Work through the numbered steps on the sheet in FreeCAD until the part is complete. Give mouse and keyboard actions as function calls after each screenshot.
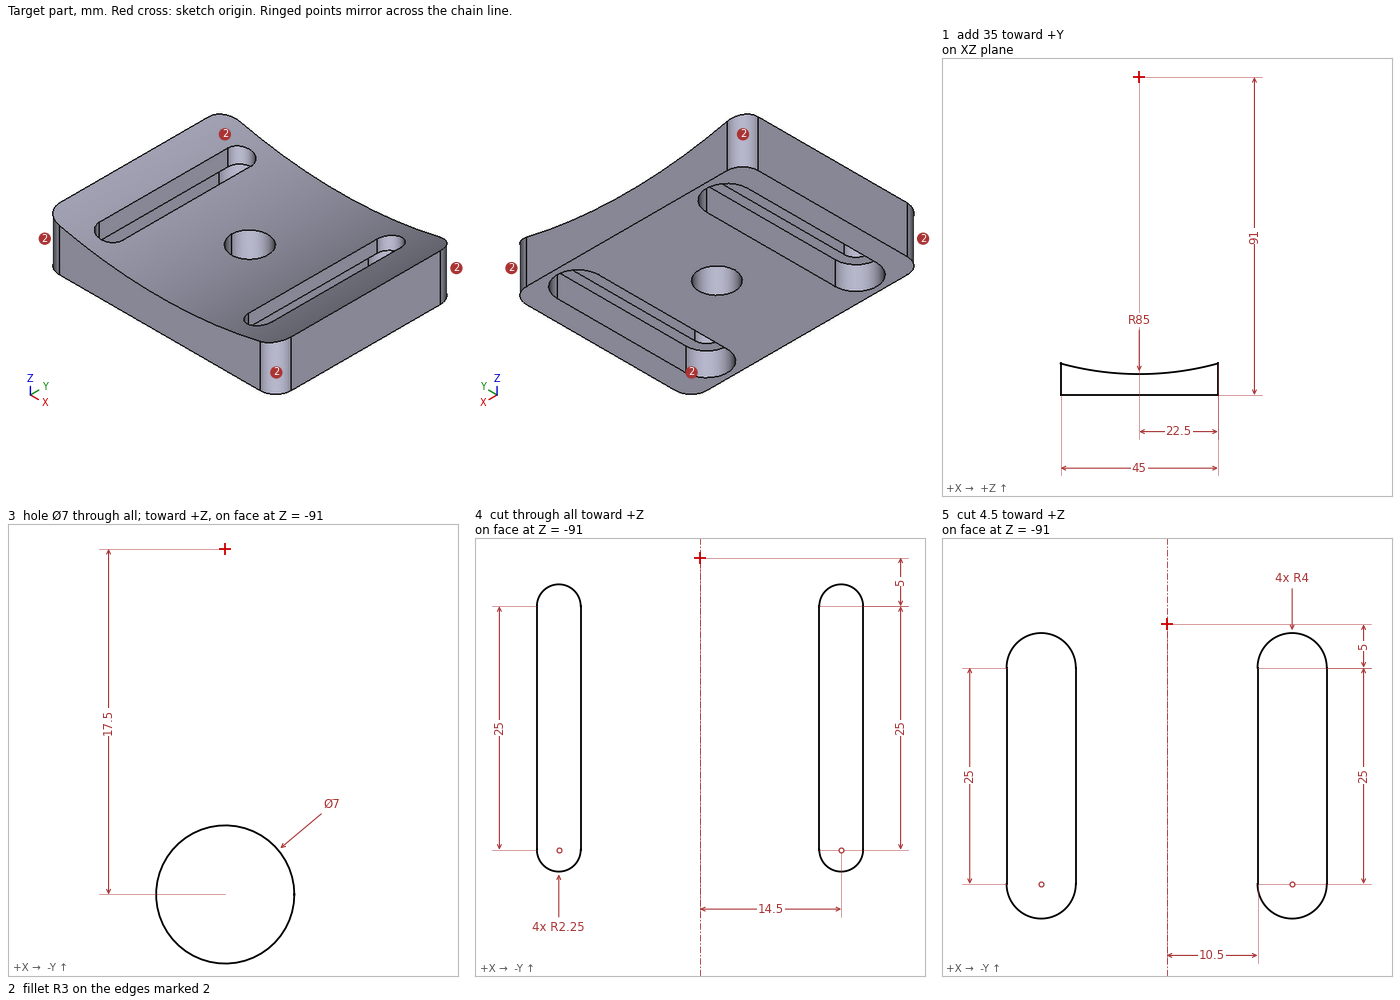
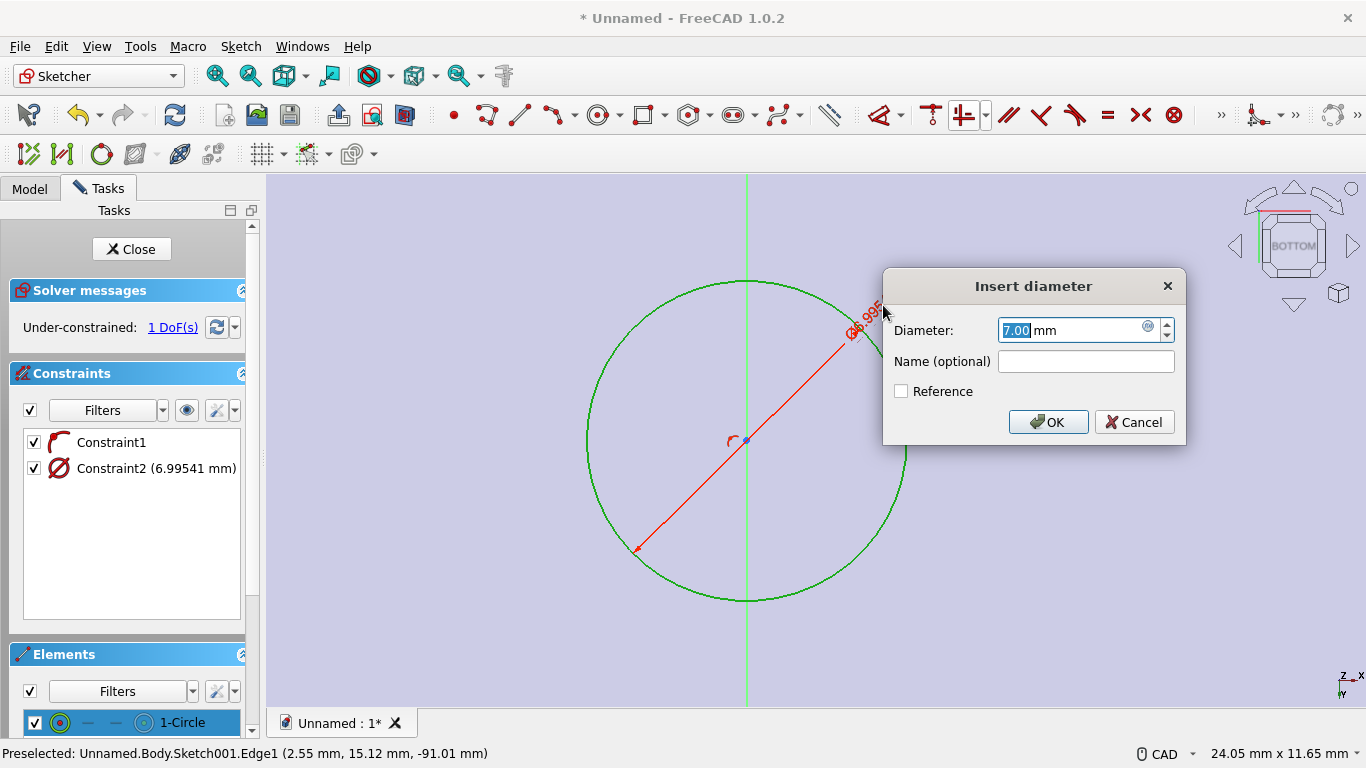
text(7)
key(Return)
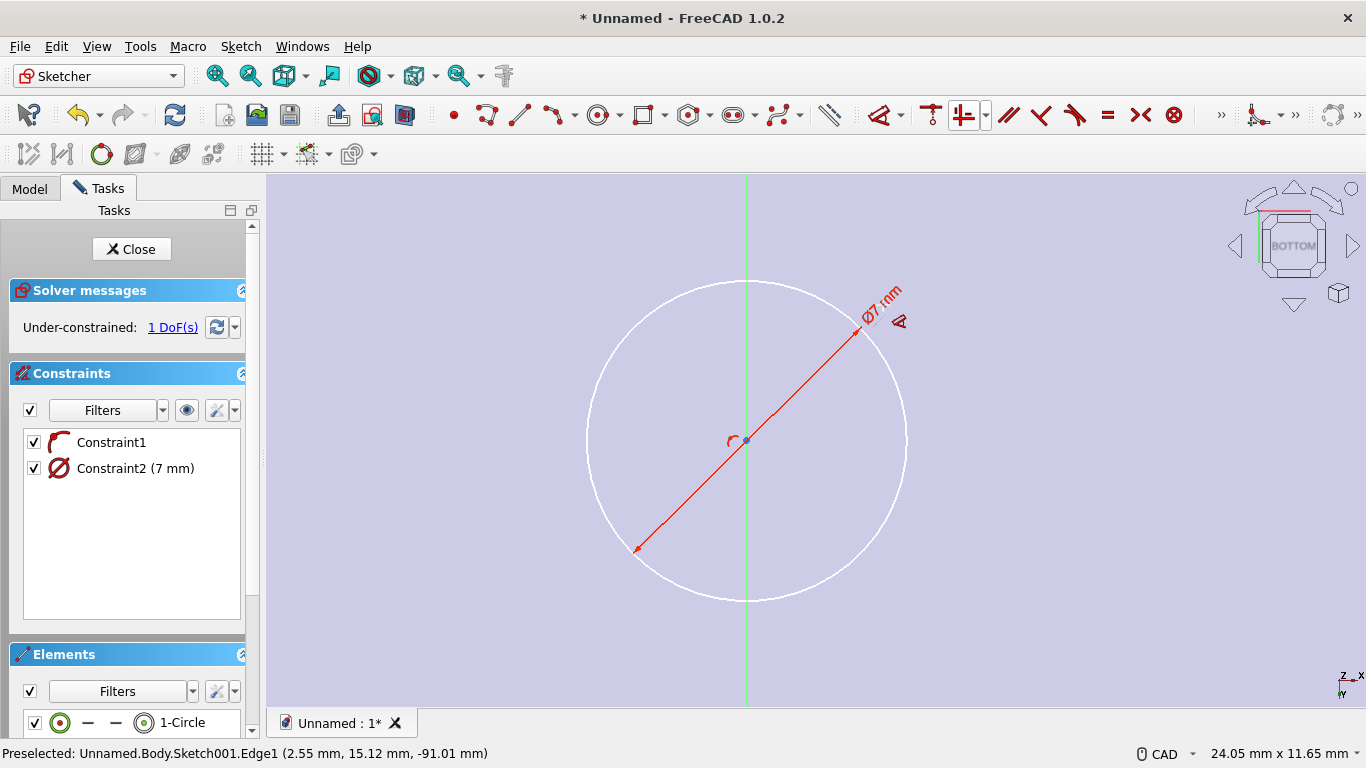
click(747, 441)
click(781, 321)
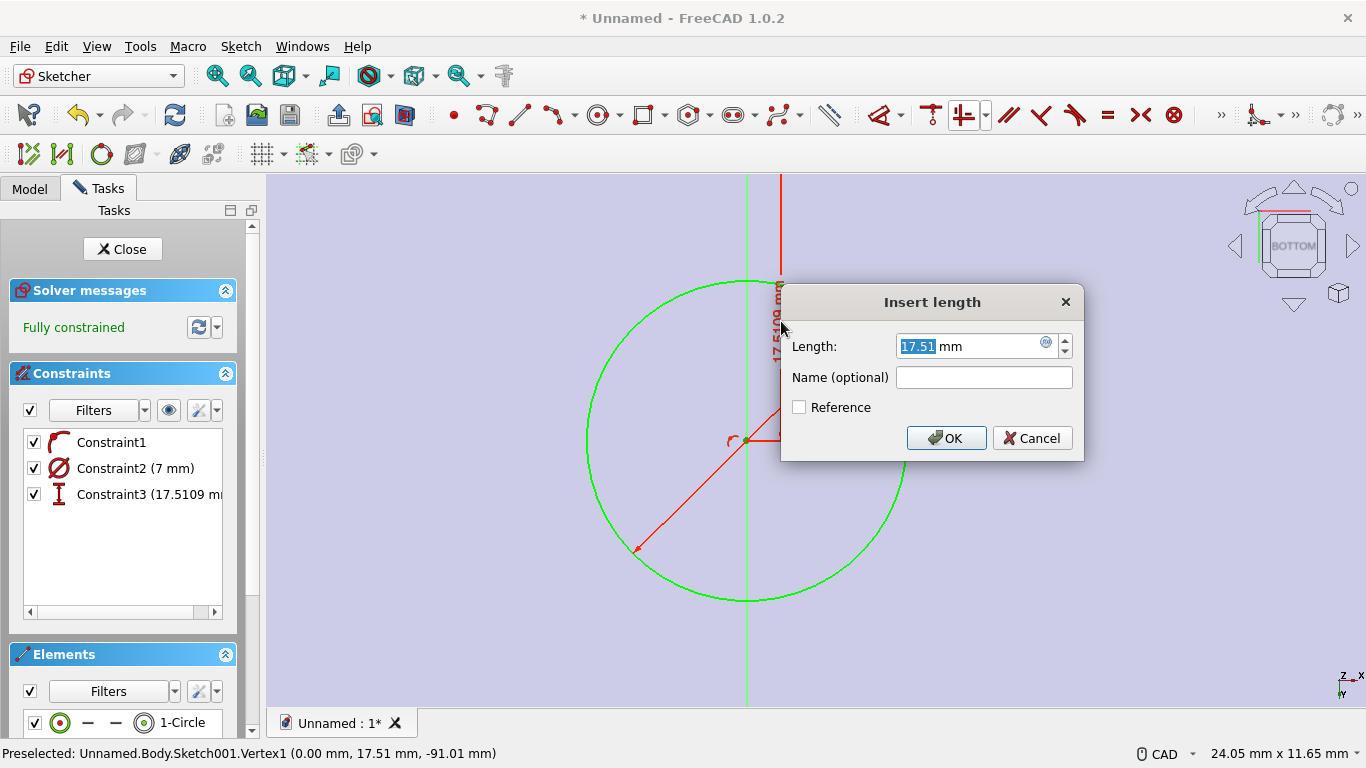
text(17.5)
key(Return)
key(Escape)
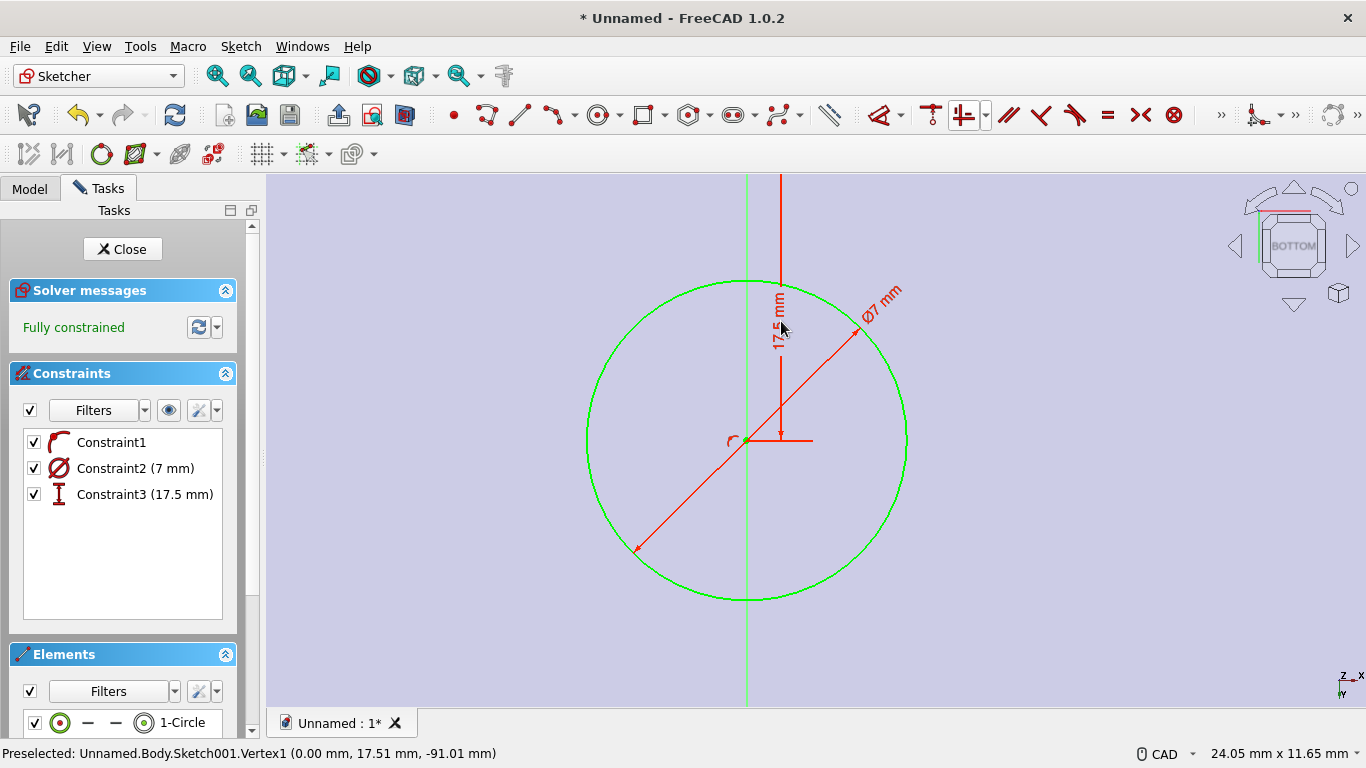
click(123, 249)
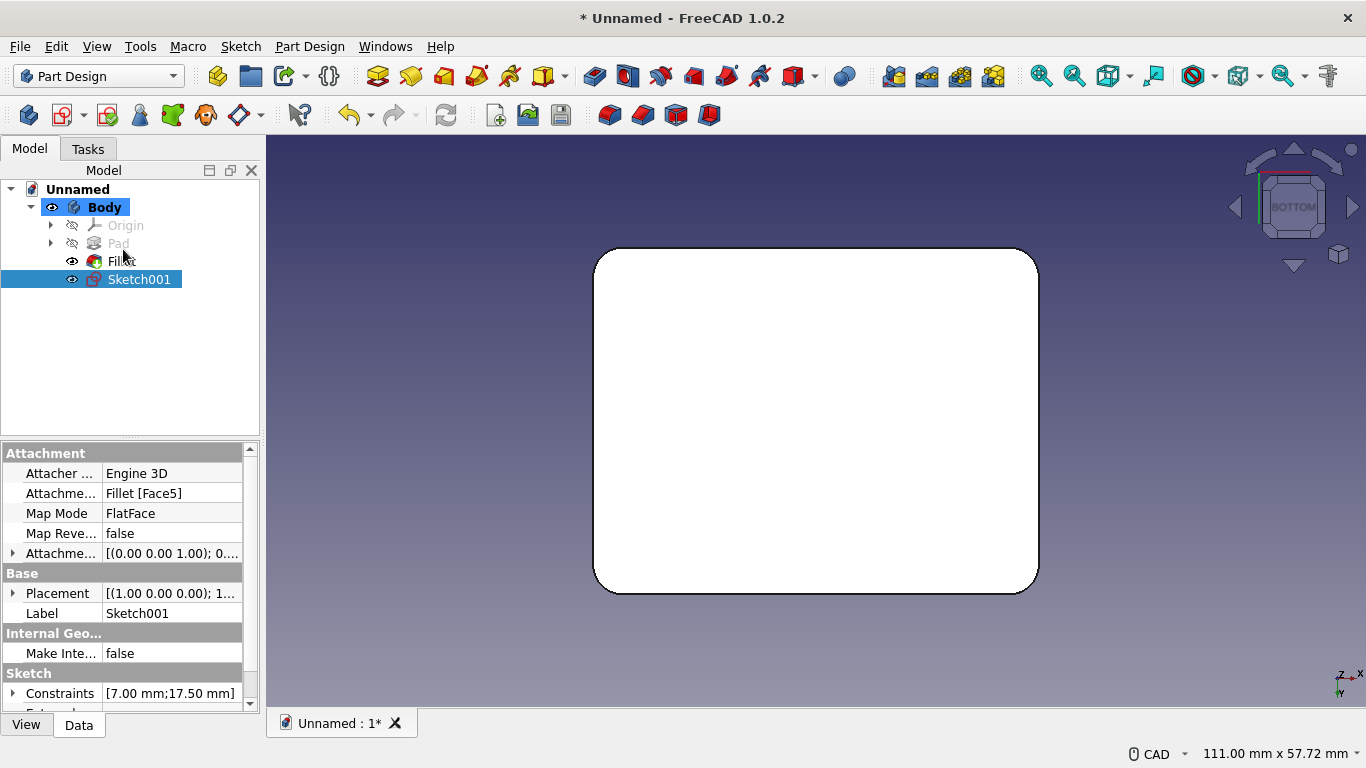
click(628, 76)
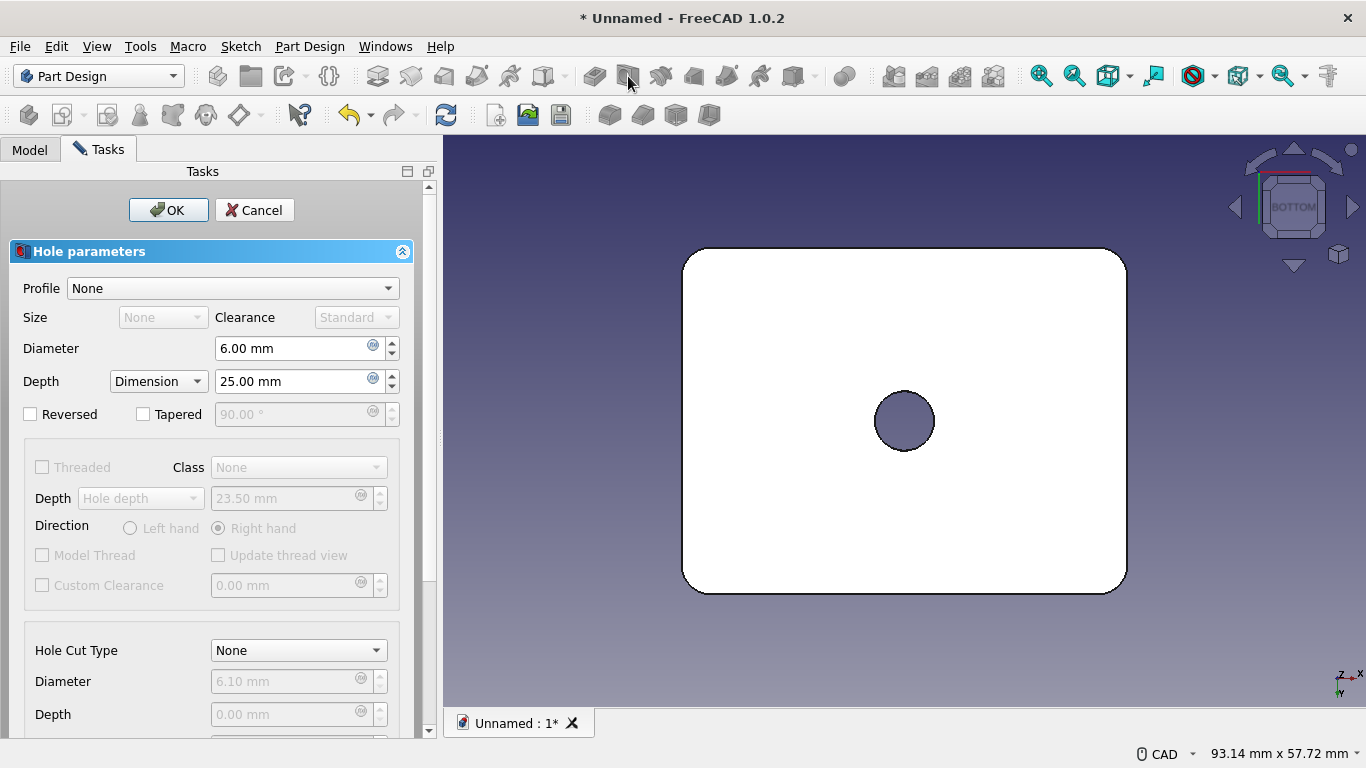
triple_click(300, 348)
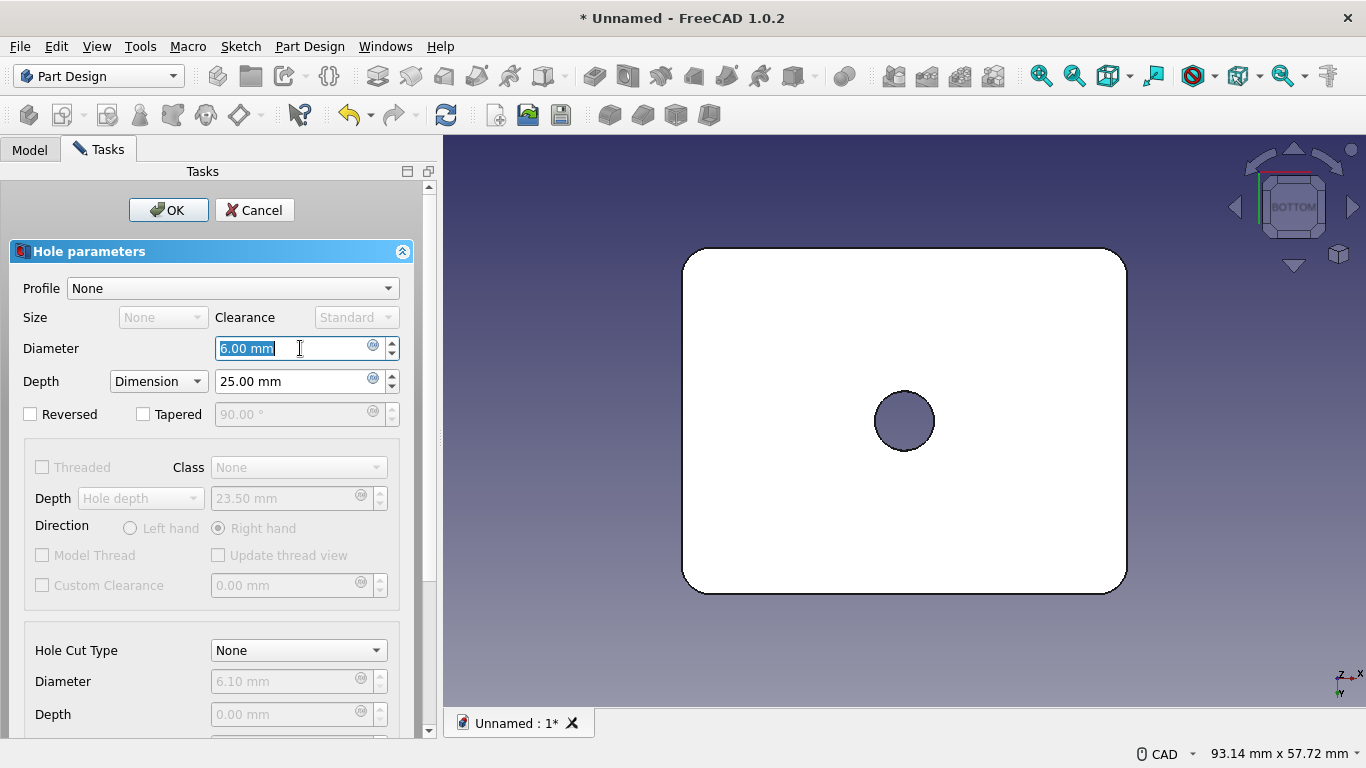
text(7)
key(Tab)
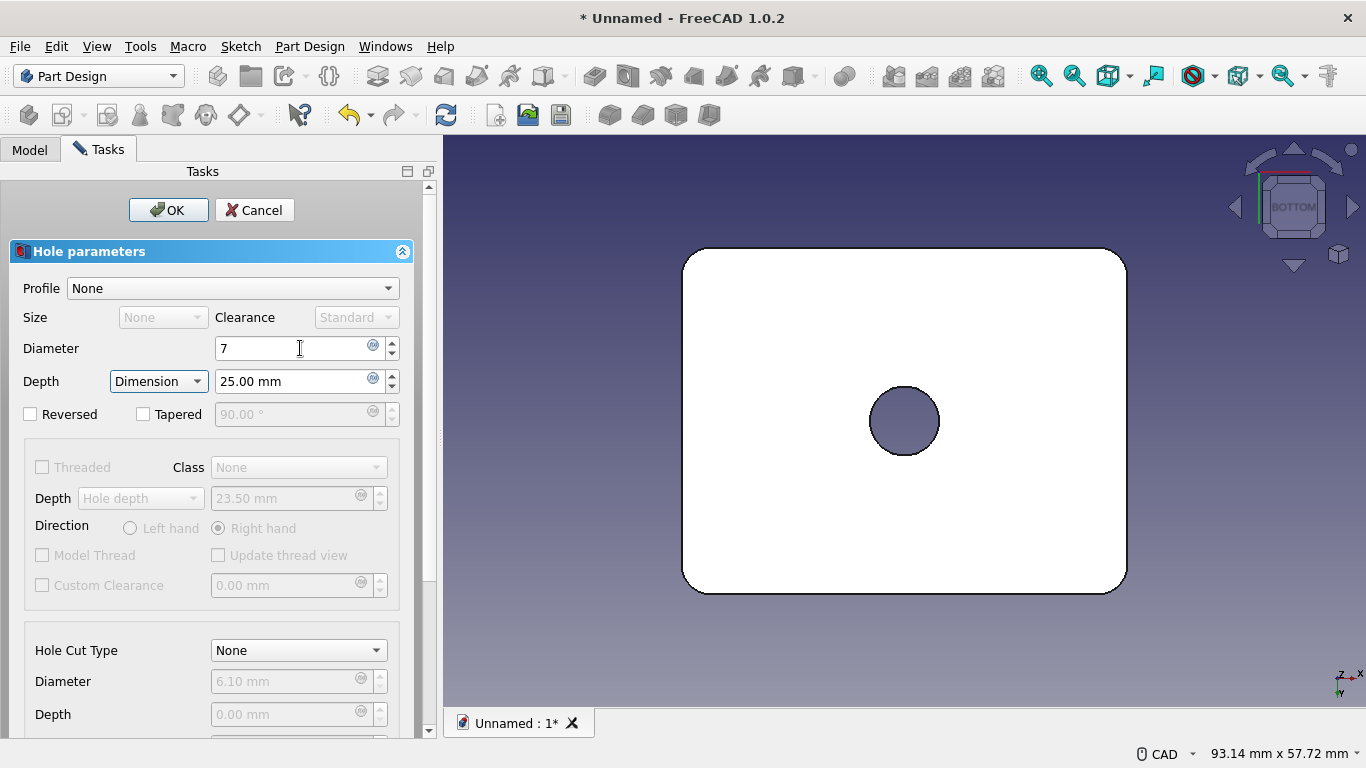
click(160, 382)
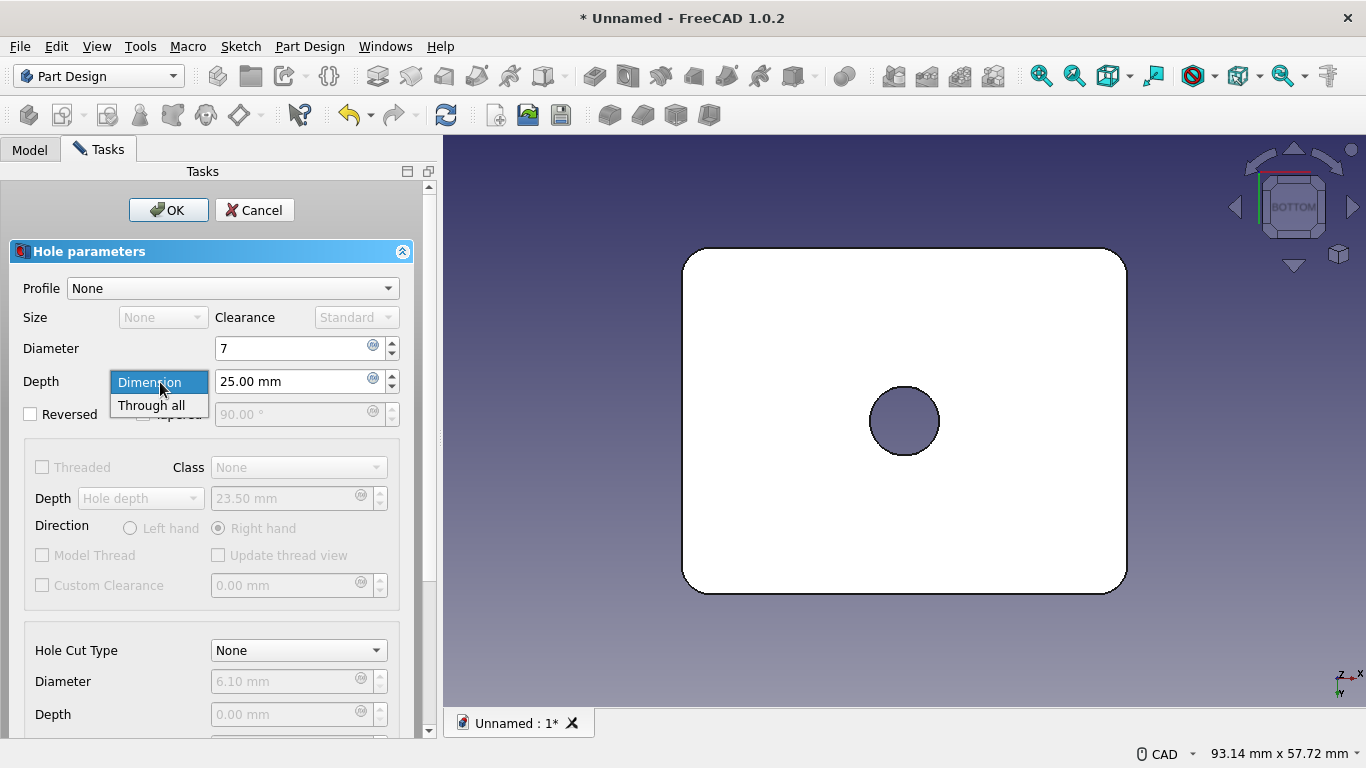
click(158, 406)